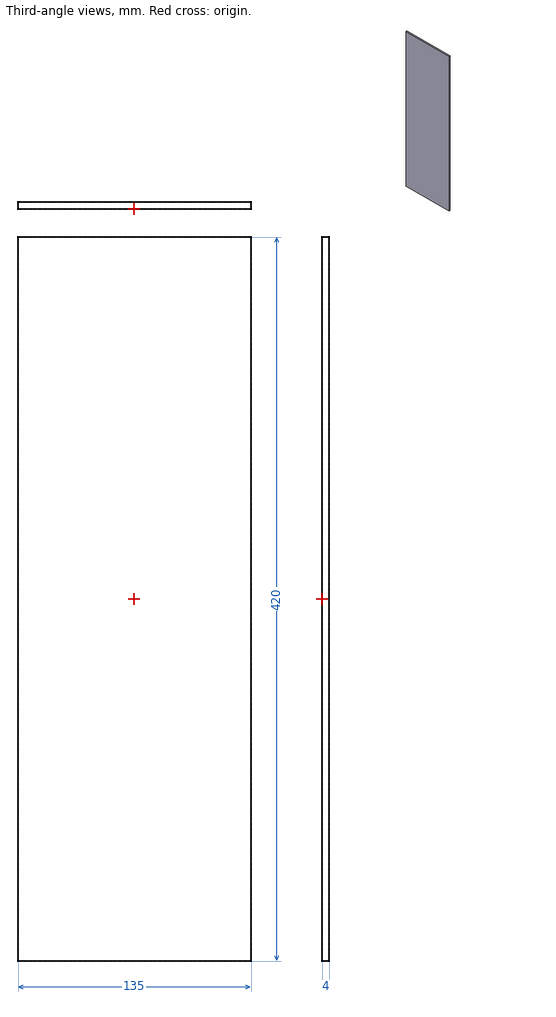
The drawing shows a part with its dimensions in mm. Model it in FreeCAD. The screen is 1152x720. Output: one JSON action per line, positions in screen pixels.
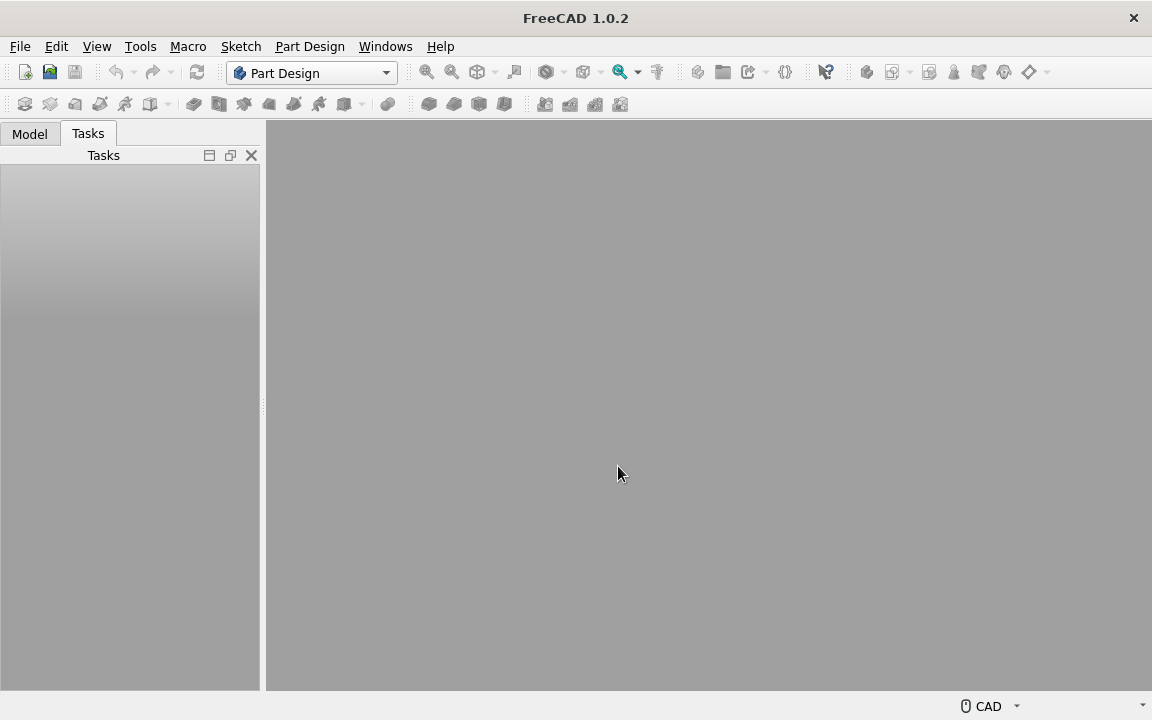
{"action": "left_click", "coordinate": [25, 72]}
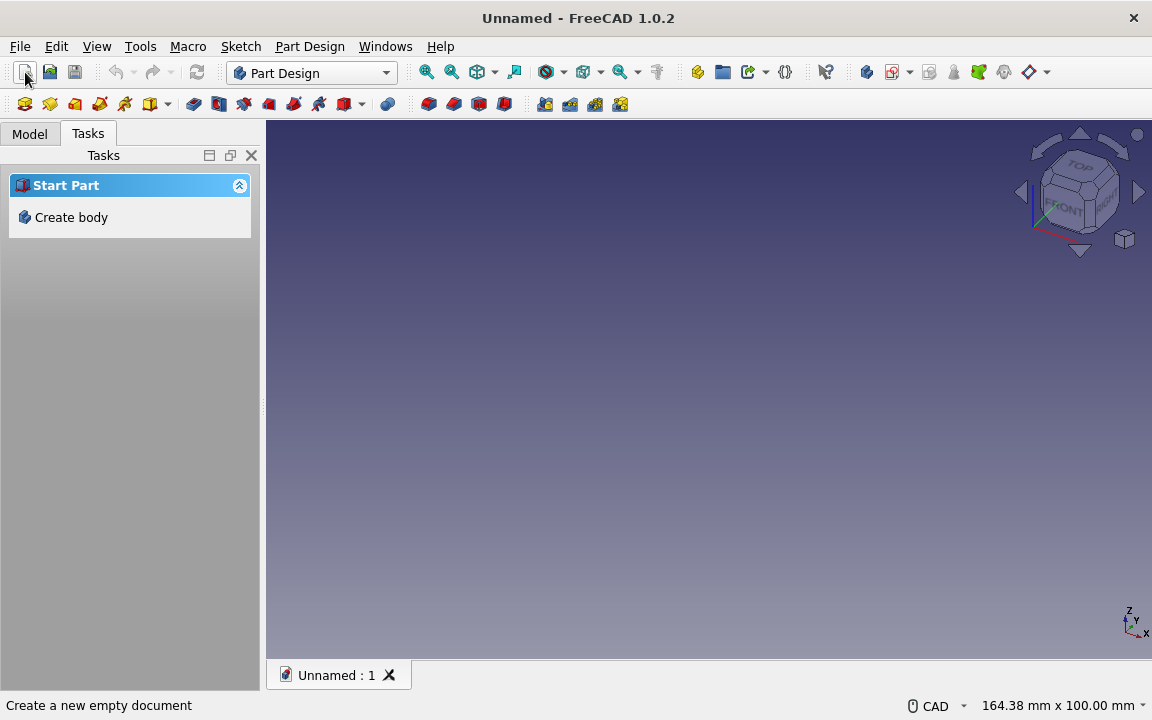
{"action": "left_click", "coordinate": [892, 72]}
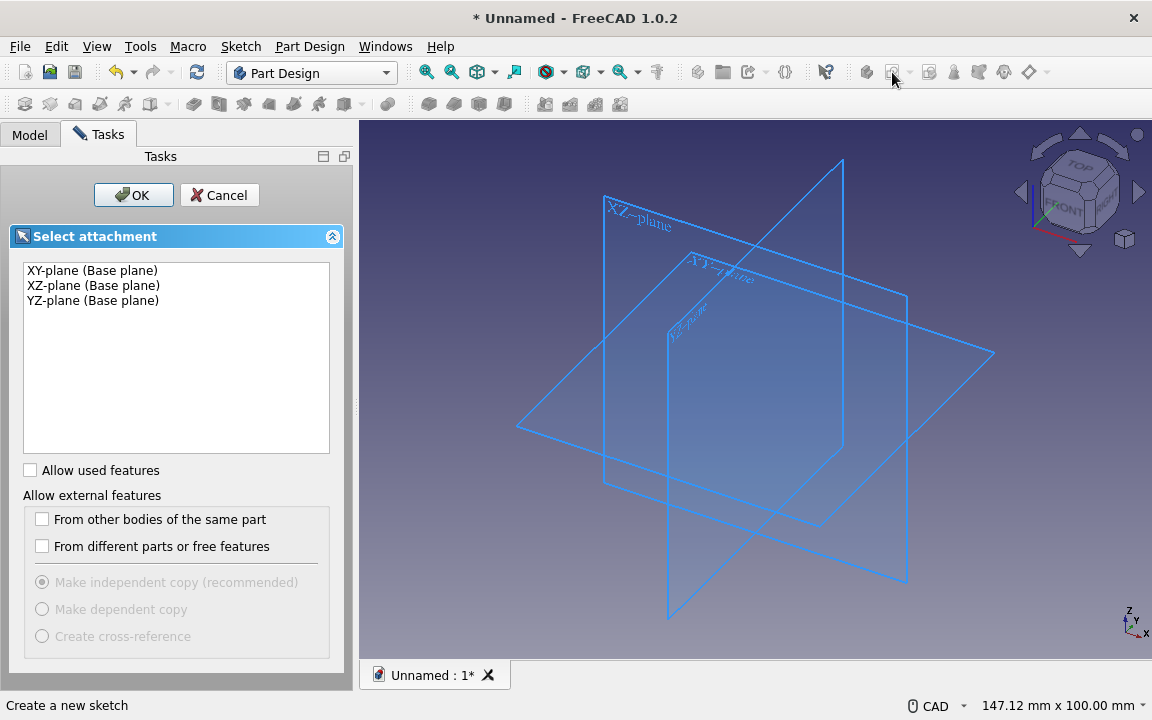
{"action": "left_click", "coordinate": [84, 286]}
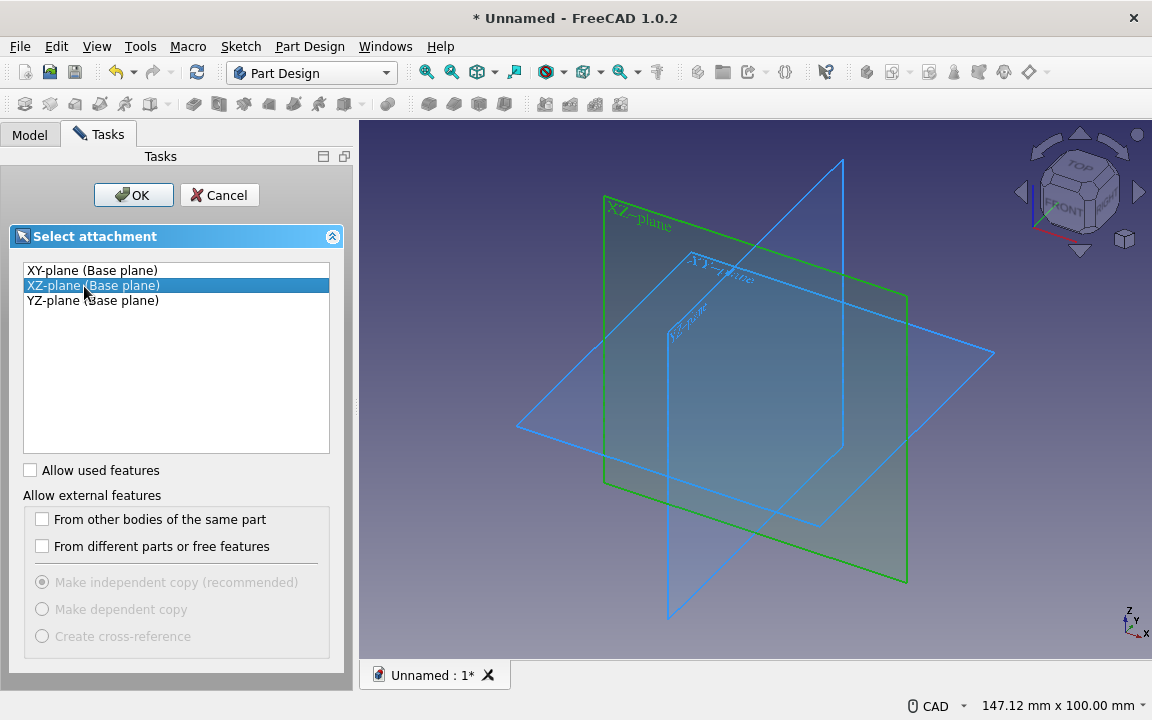
{"action": "left_click", "coordinate": [134, 195]}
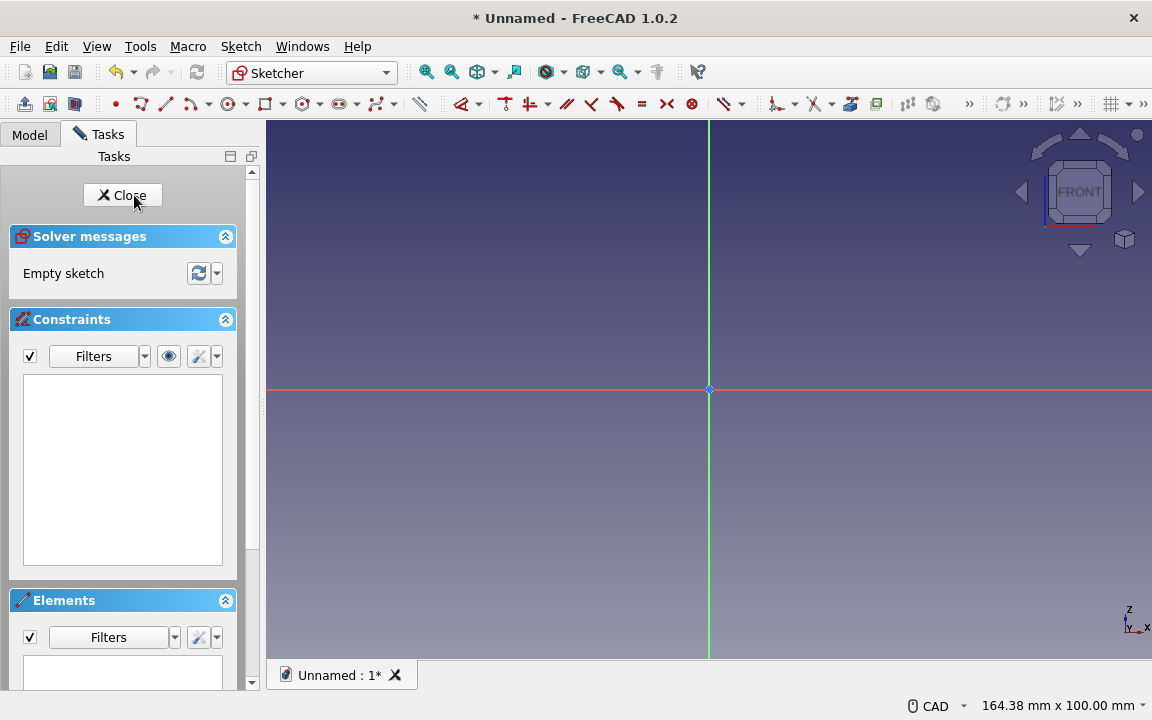
{"action": "scroll", "coordinate": [627, 390], "scroll_direction": "down", "scroll_amount": 9}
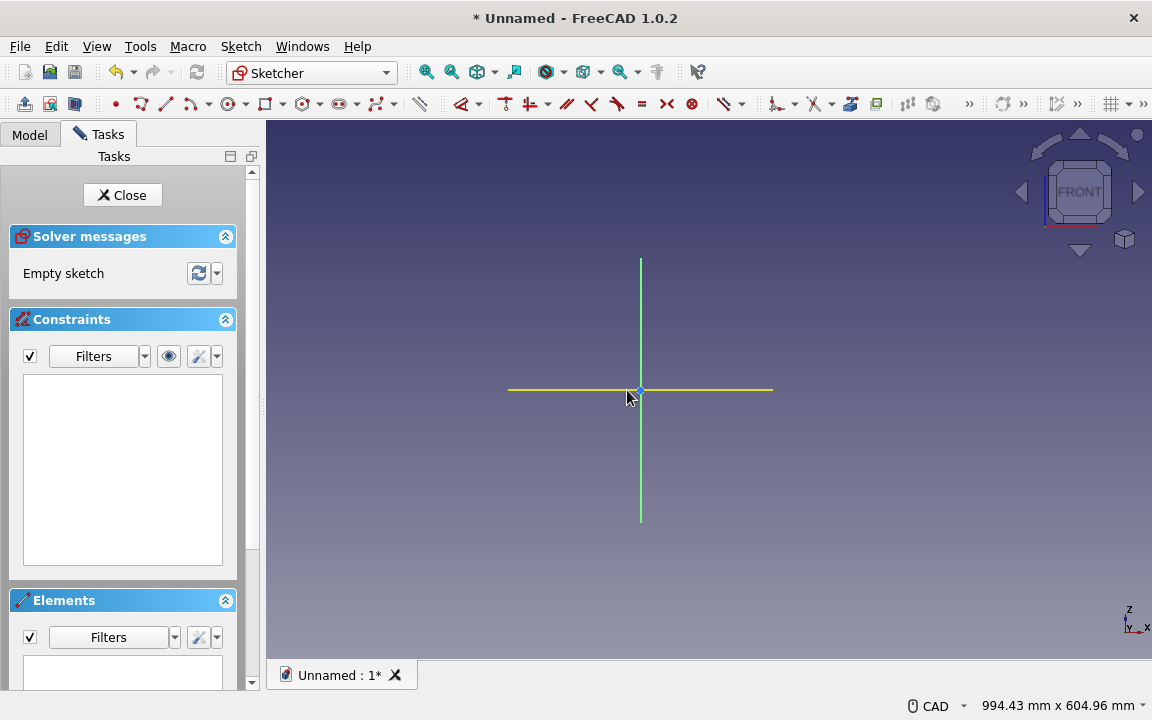
{"action": "key", "text": "g v"}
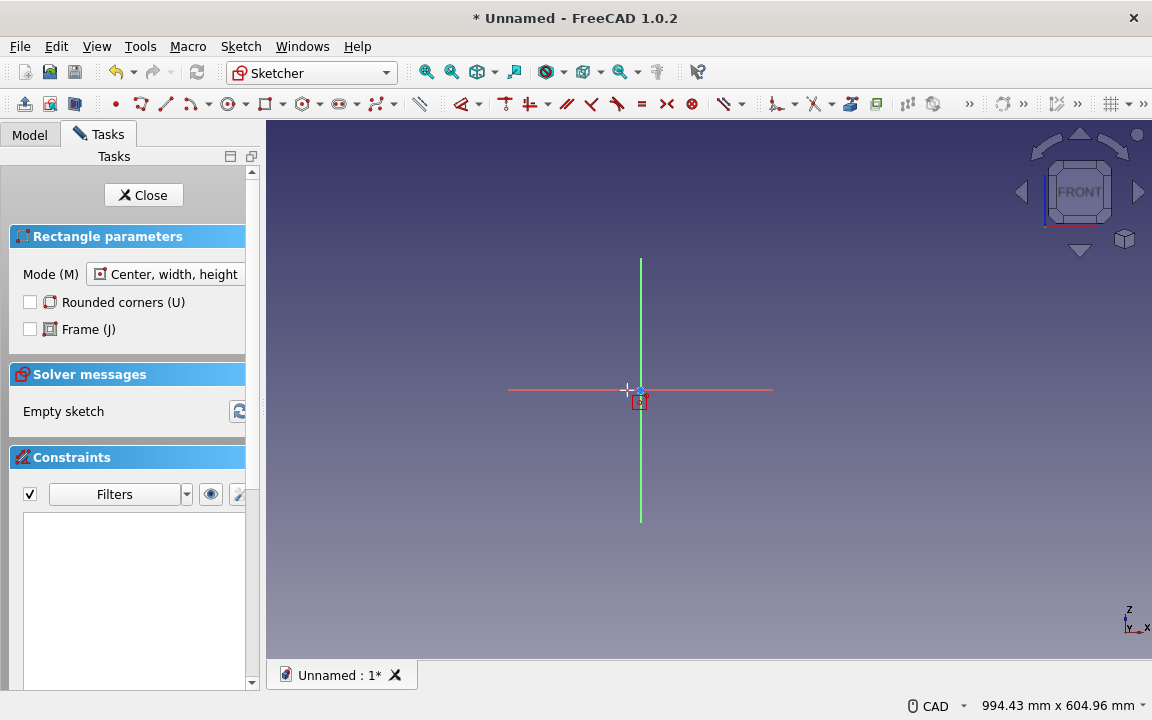
{"action": "left_click", "coordinate": [641, 390]}
{"action": "mouse_move", "coordinate": [701, 203]}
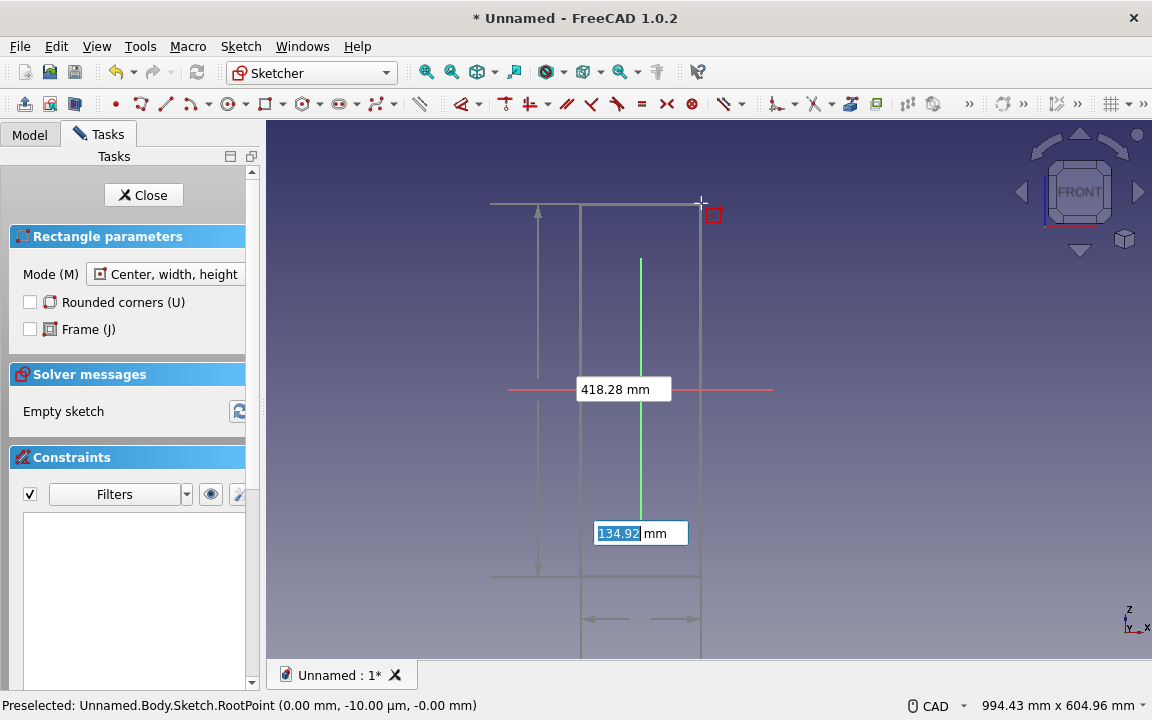
{"action": "type", "text": "135"}
{"action": "key", "text": "Tab"}
{"action": "type", "text": "420"}
{"action": "key", "text": "Return"}
{"action": "key", "text": "Escape"}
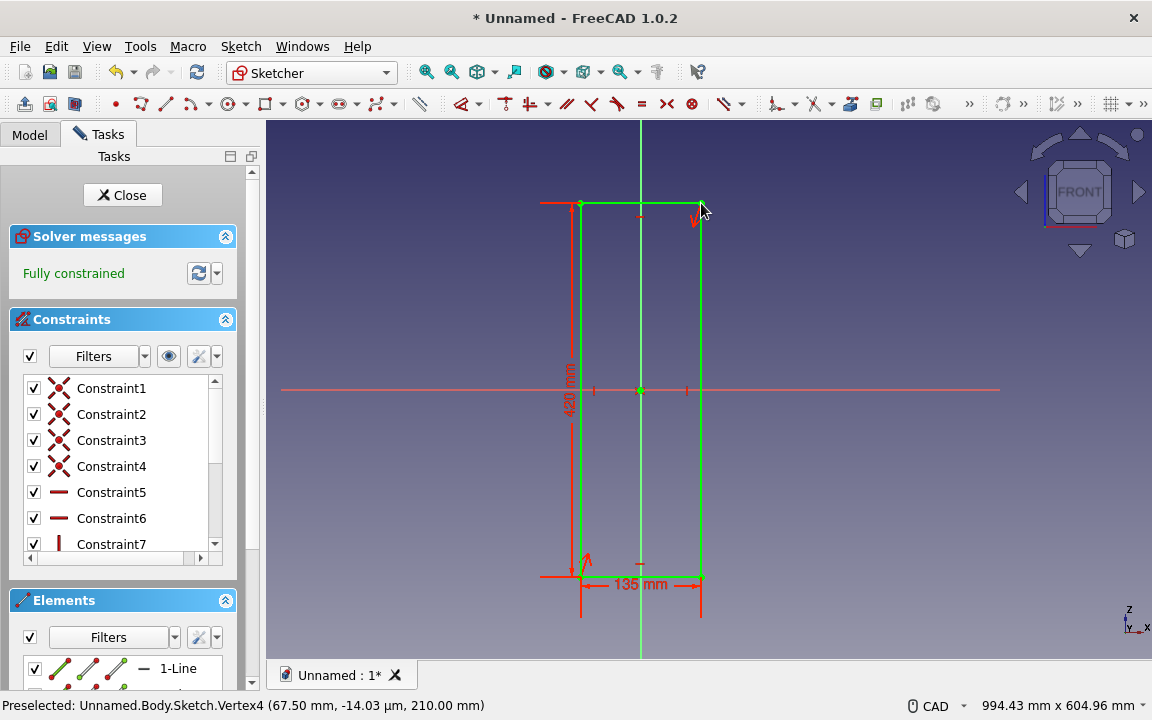
{"action": "left_click", "coordinate": [123, 195]}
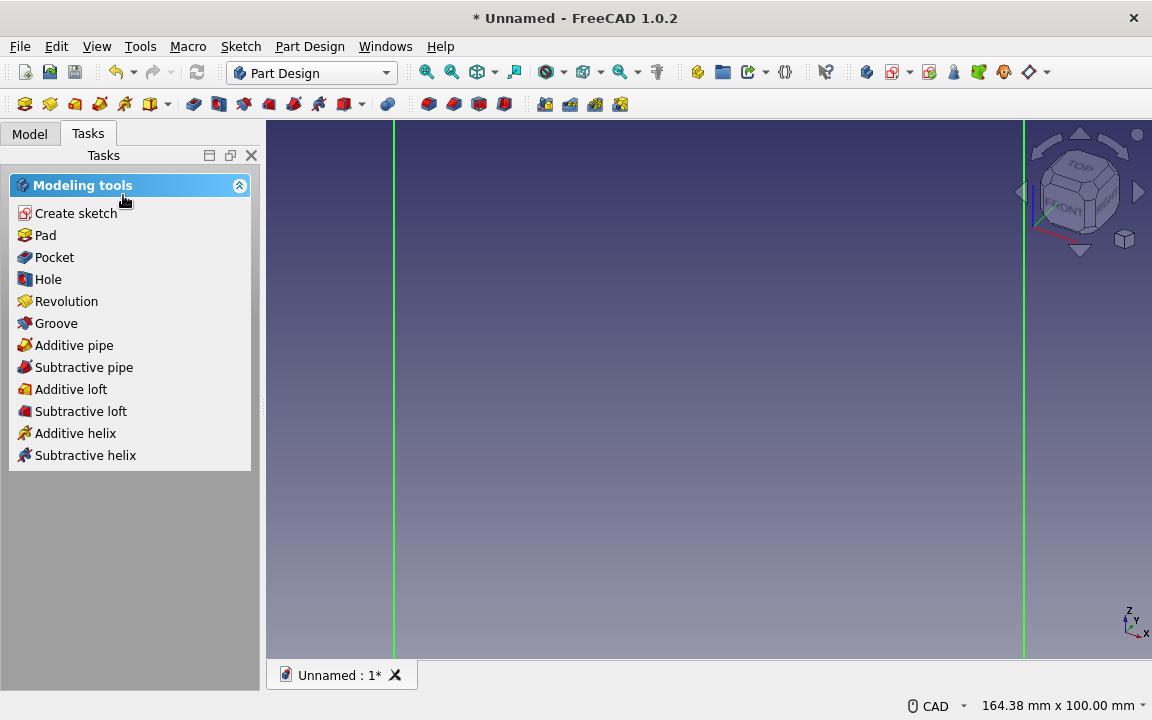
{"action": "left_click", "coordinate": [25, 104]}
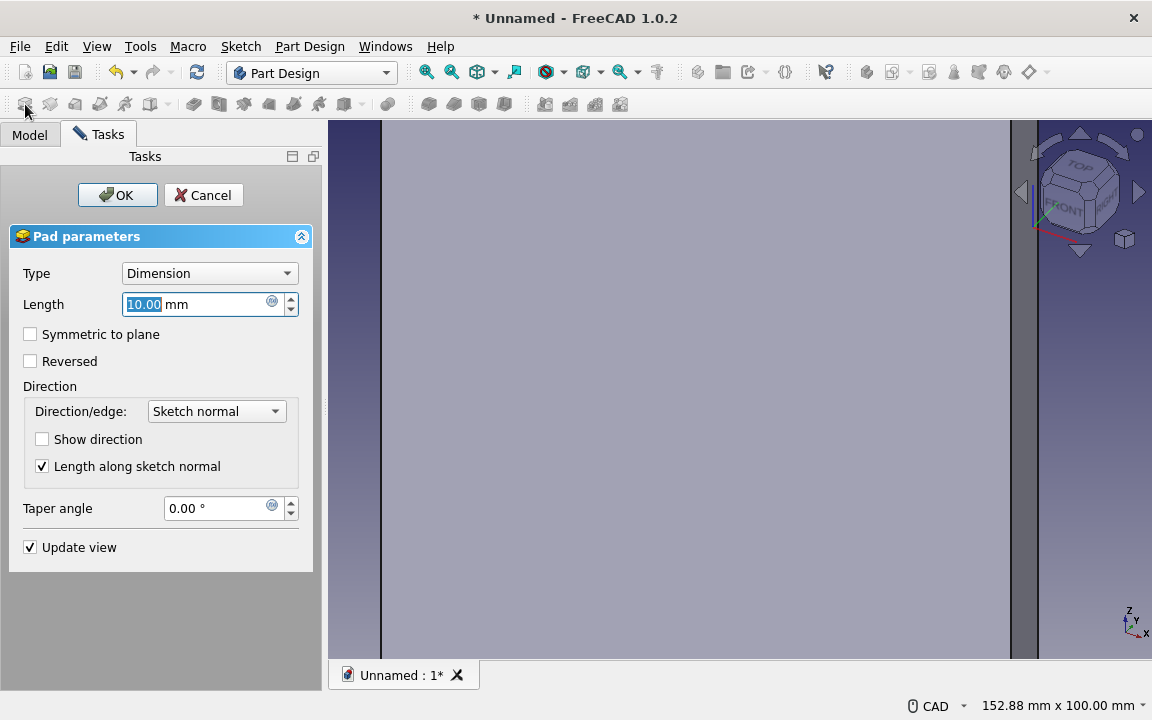
{"action": "type", "text": "4"}
{"action": "key", "text": "Tab"}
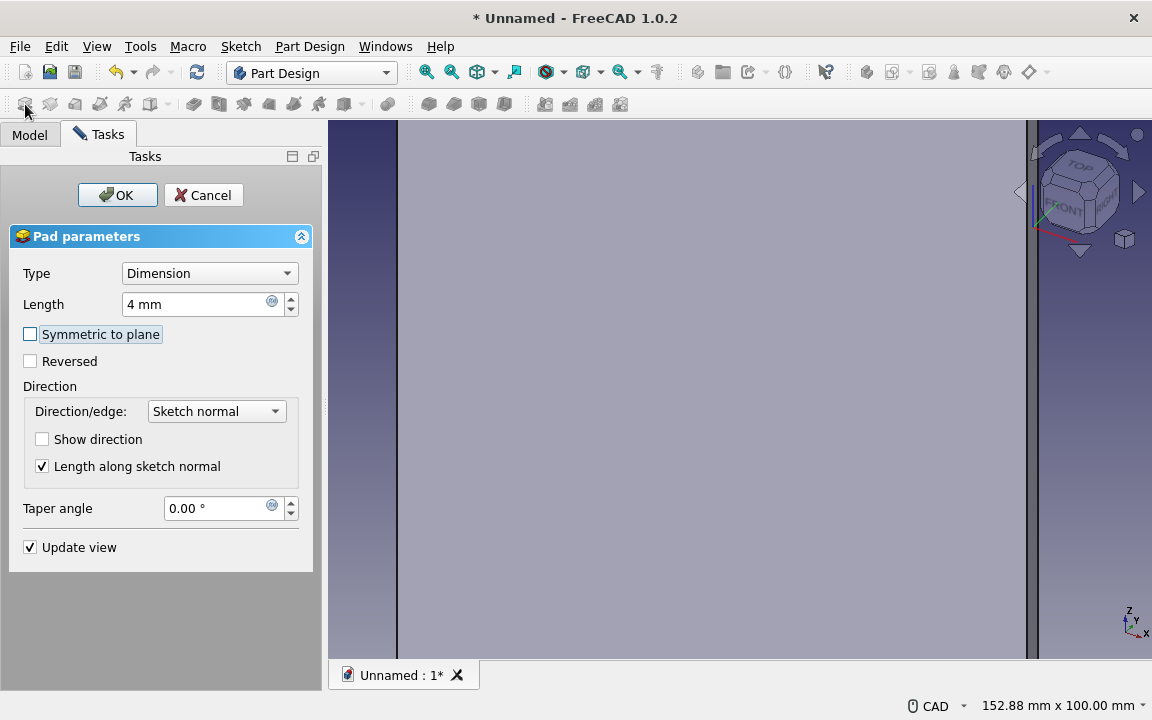
{"action": "left_click", "coordinate": [31, 361]}